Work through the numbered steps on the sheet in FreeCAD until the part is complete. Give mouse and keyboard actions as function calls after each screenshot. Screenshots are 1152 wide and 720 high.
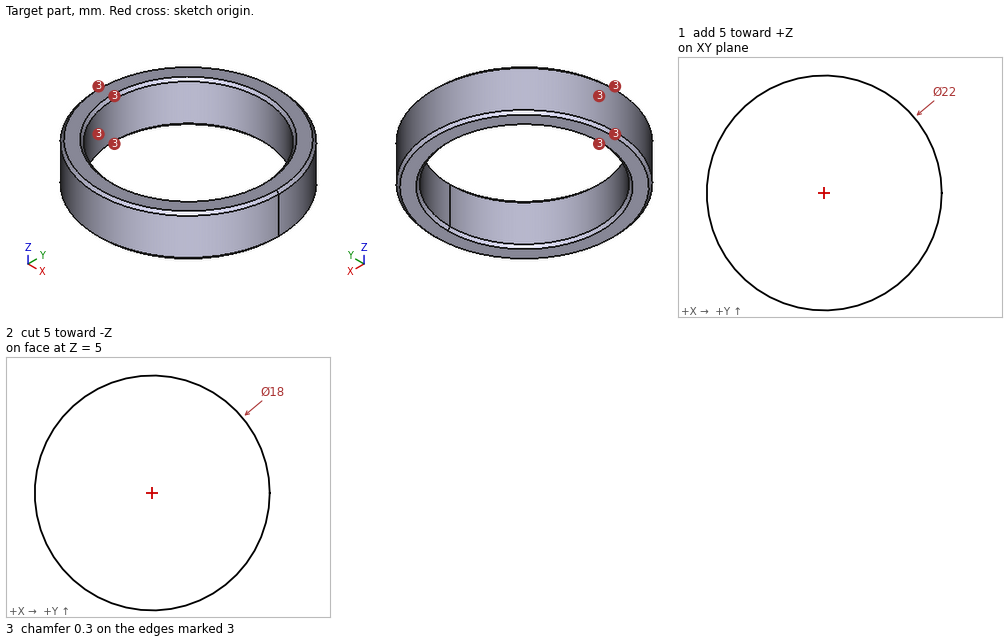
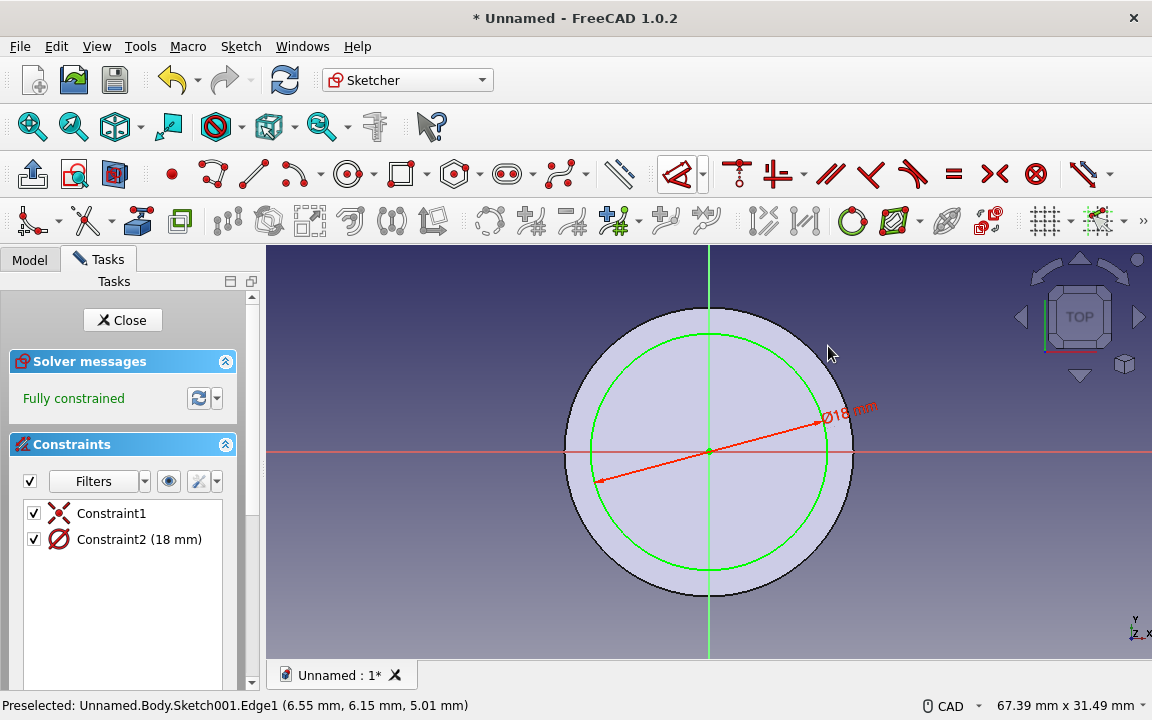
click(123, 320)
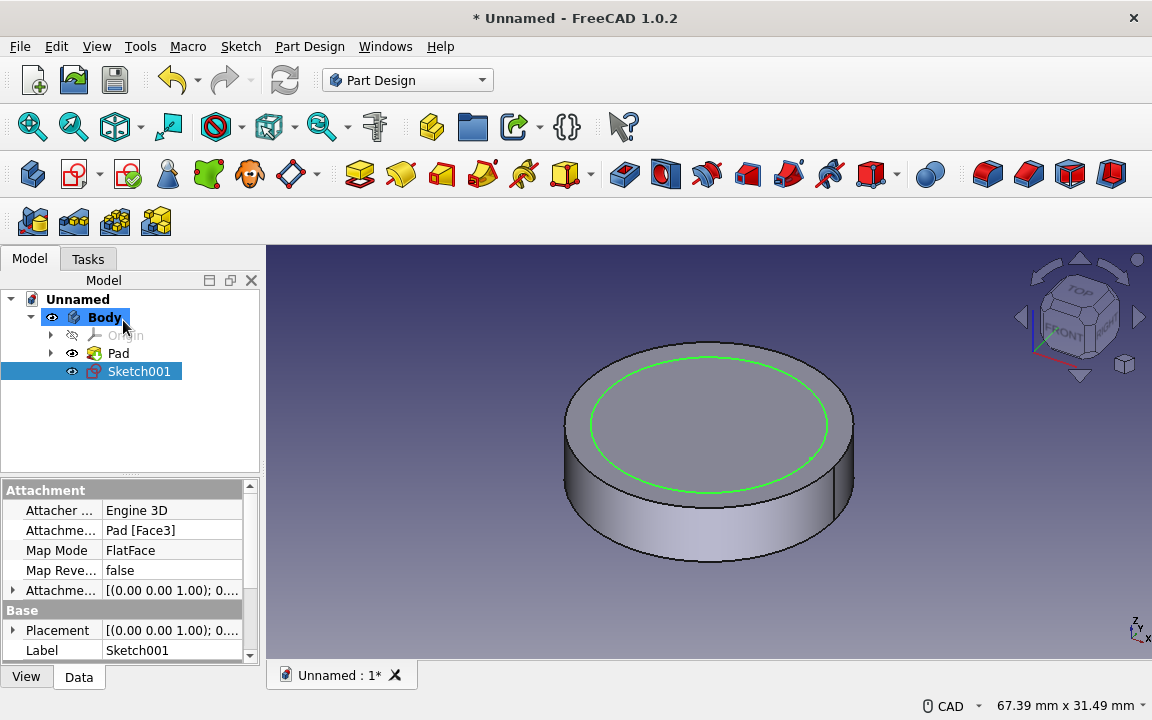
click(625, 174)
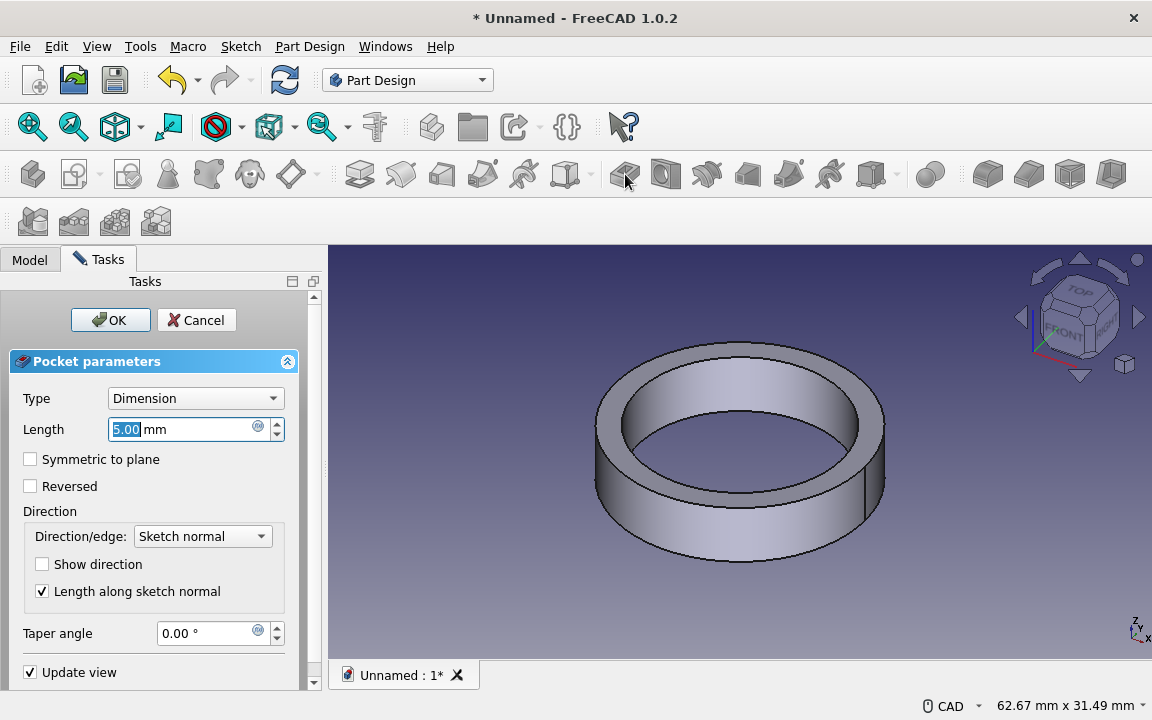
text(5)
key(Tab)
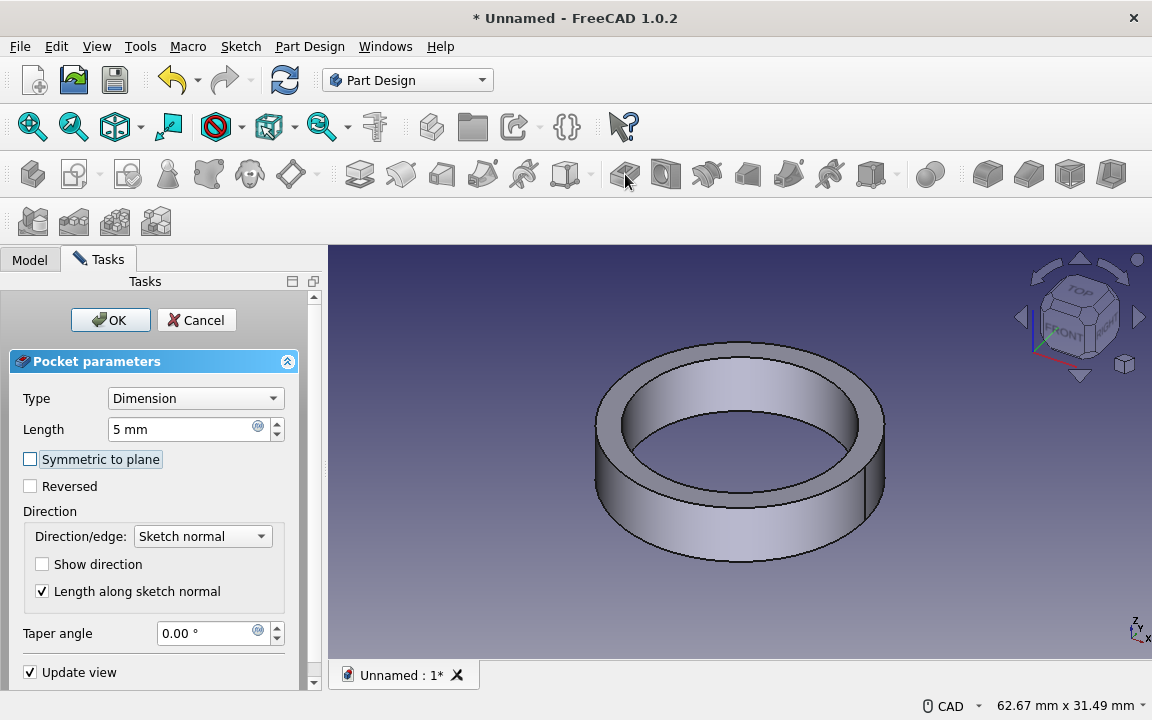
click(111, 320)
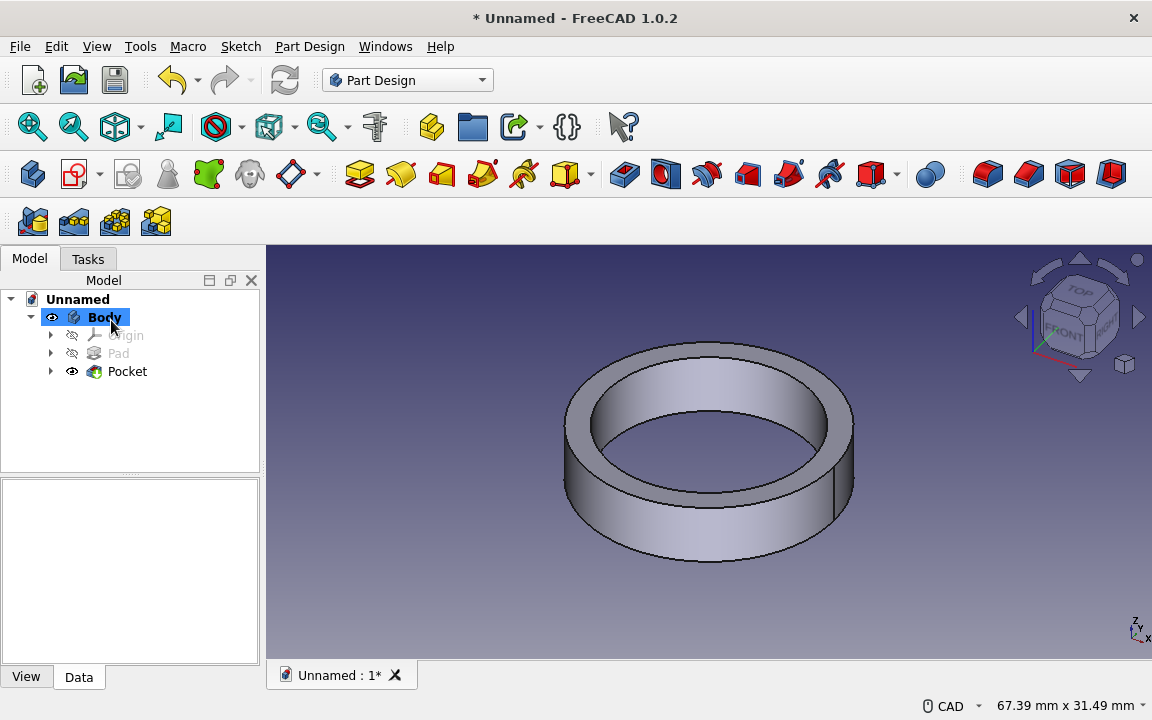
click(565, 433)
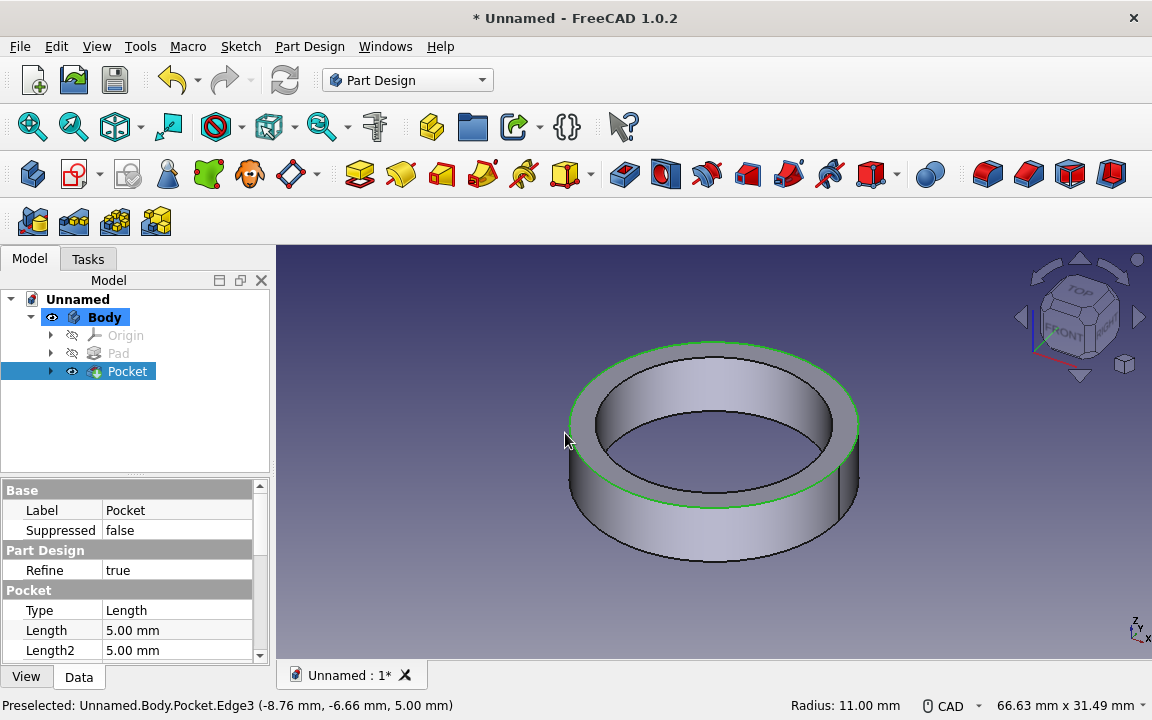
click(612, 390, ctrl)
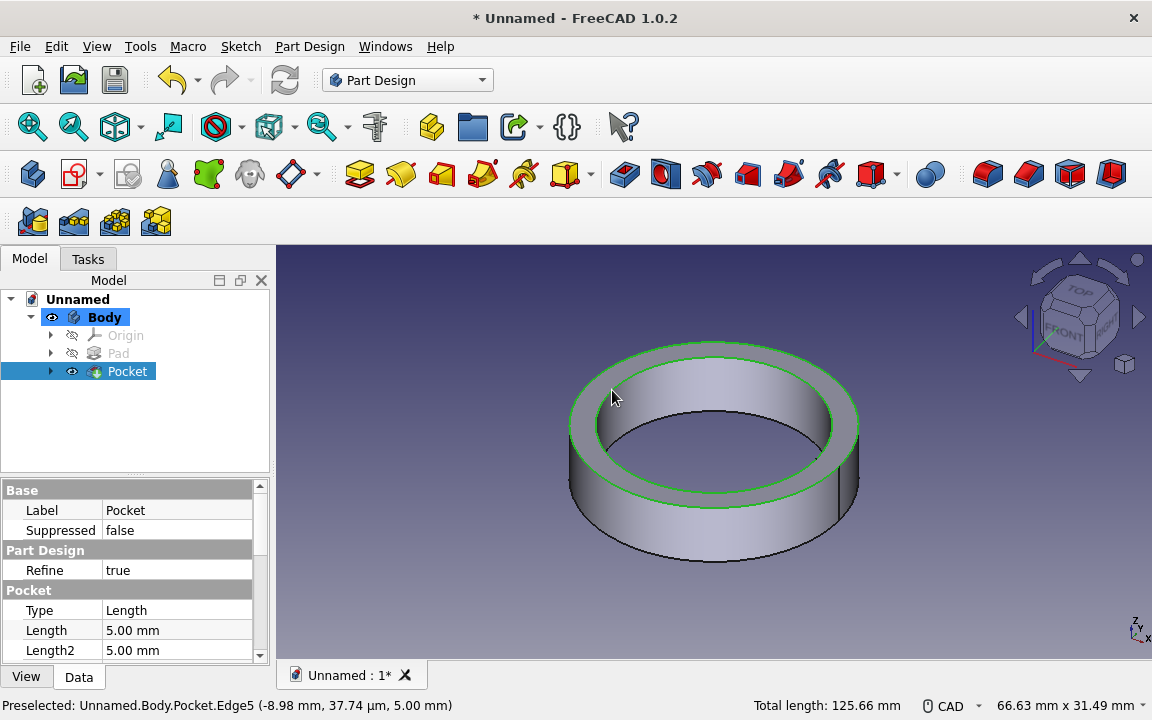
key(0)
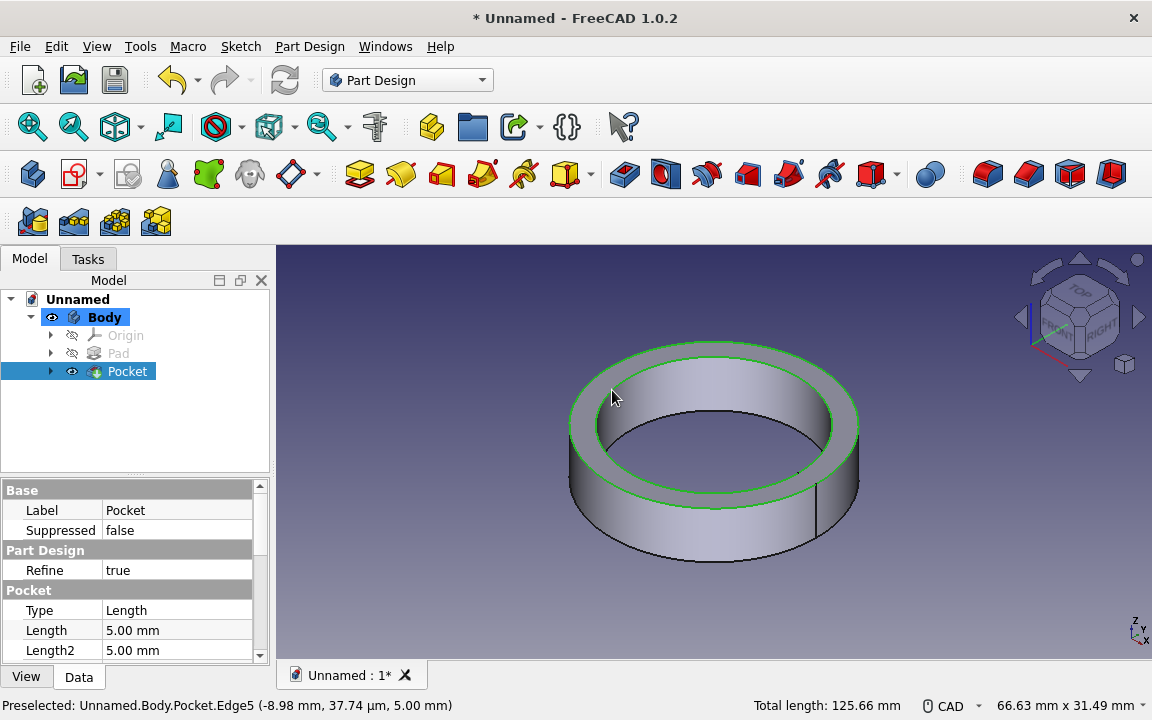
key(2)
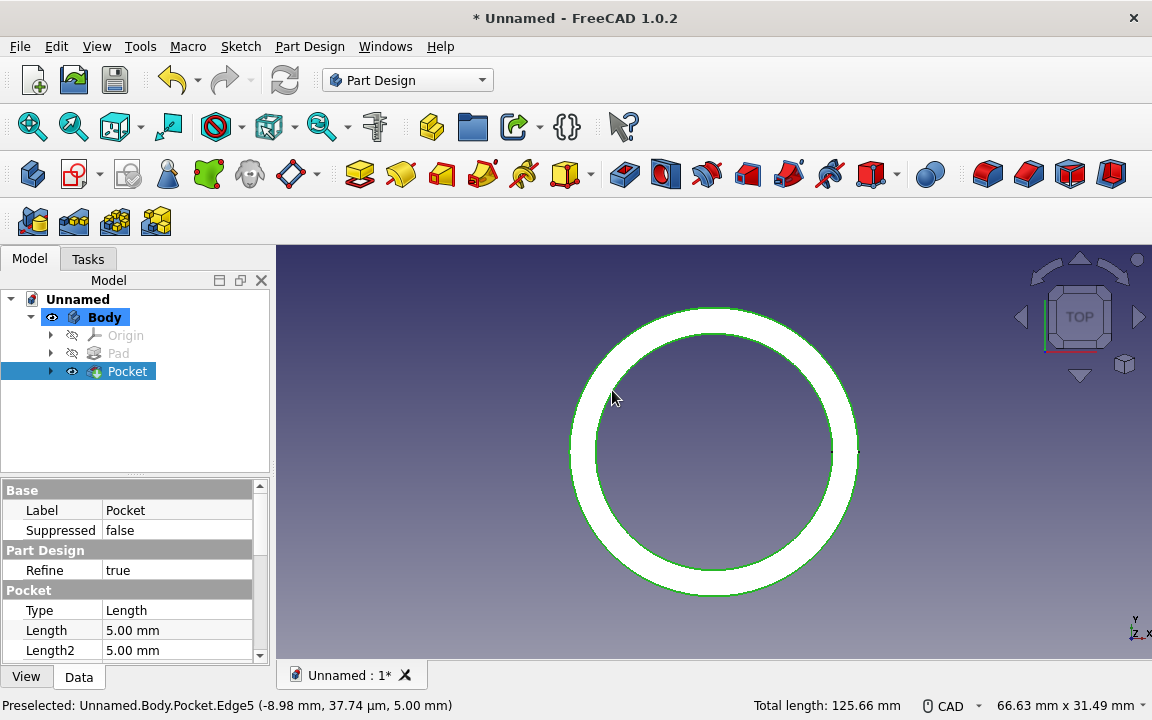
key(1)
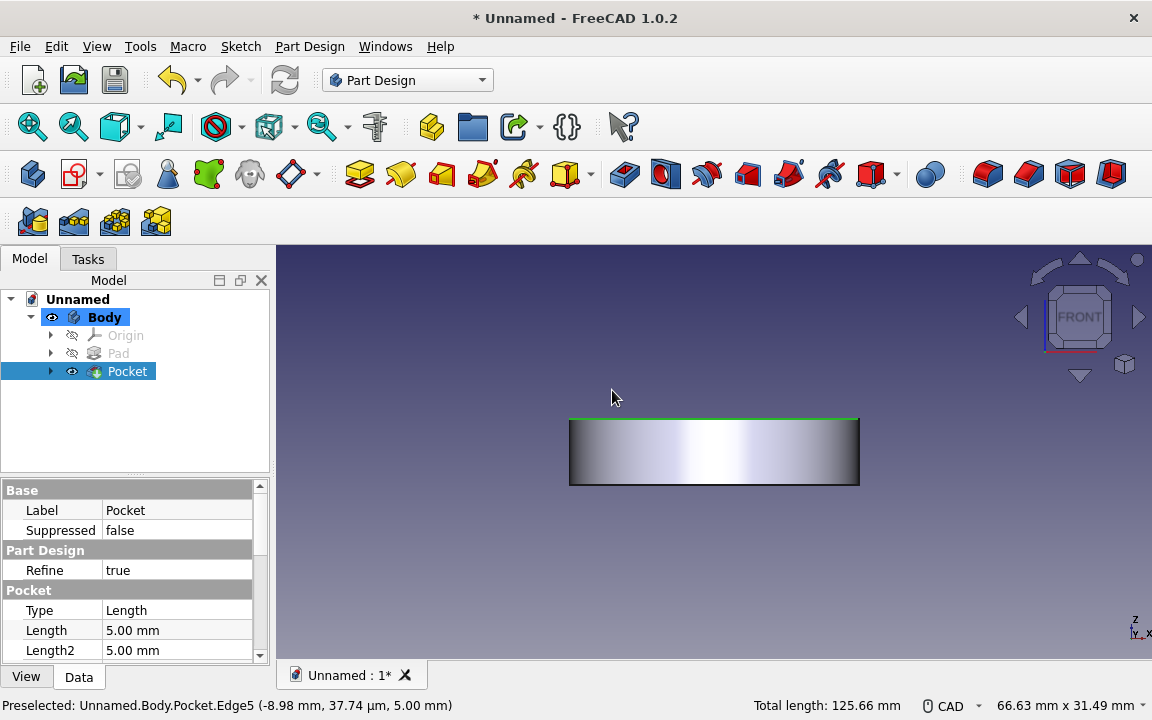
click(33, 128)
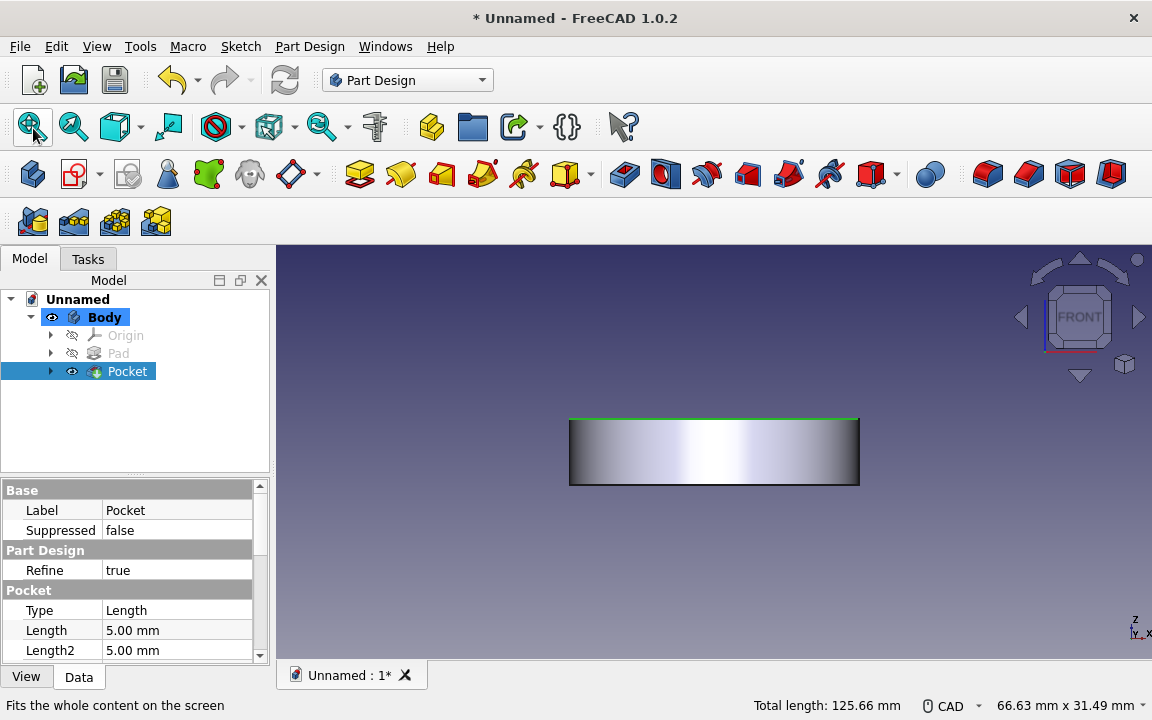
click(597, 484, ctrl)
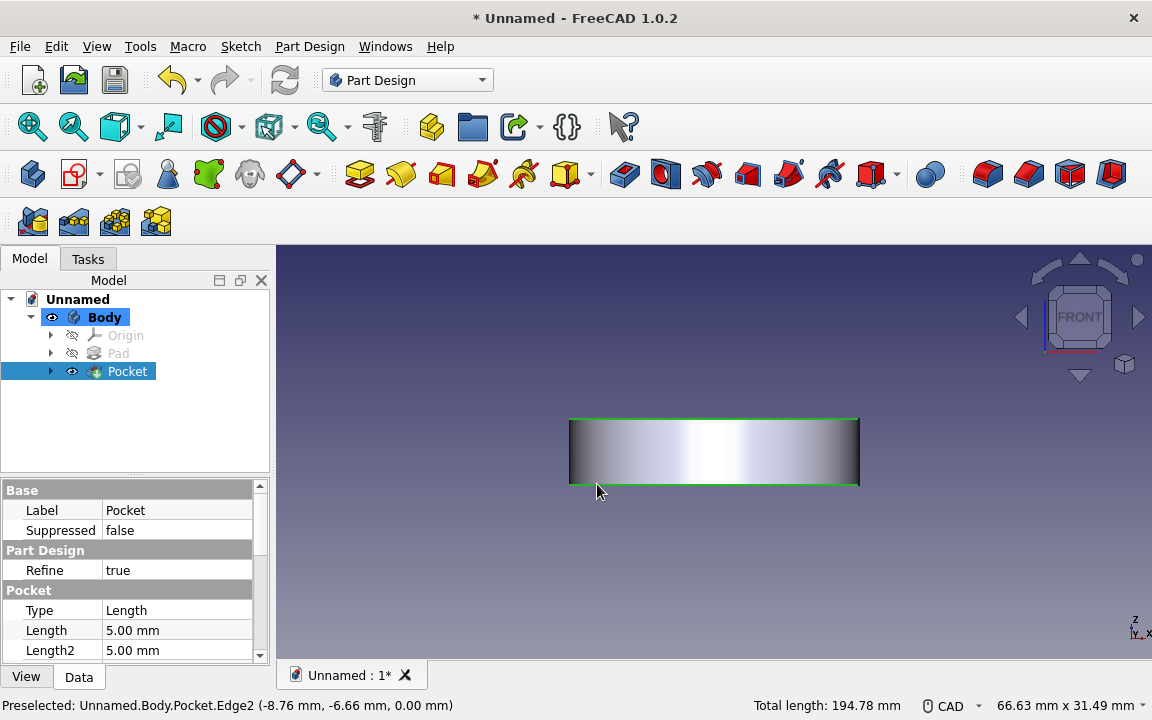
key(3)